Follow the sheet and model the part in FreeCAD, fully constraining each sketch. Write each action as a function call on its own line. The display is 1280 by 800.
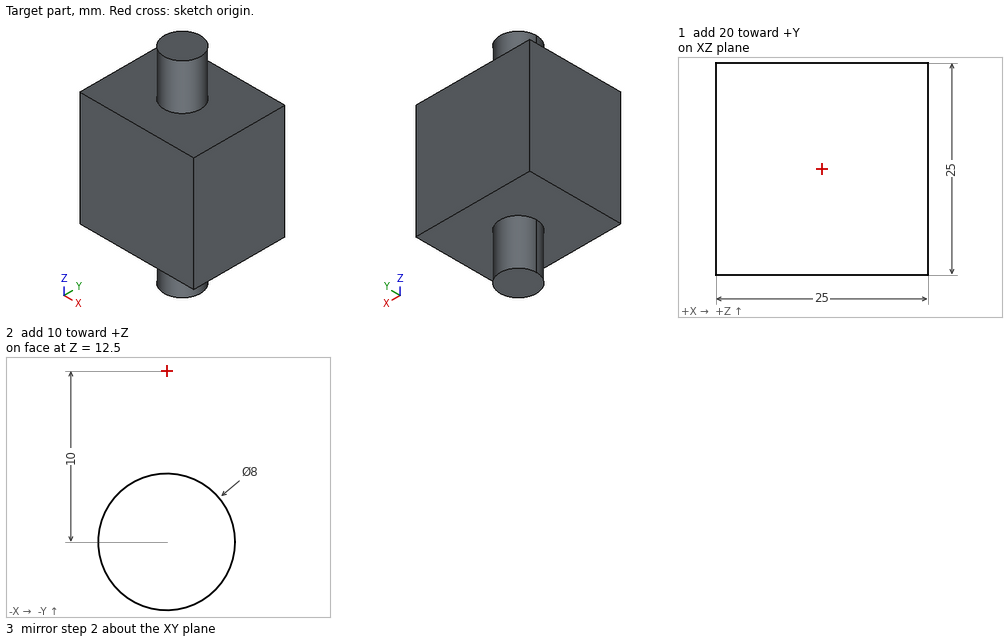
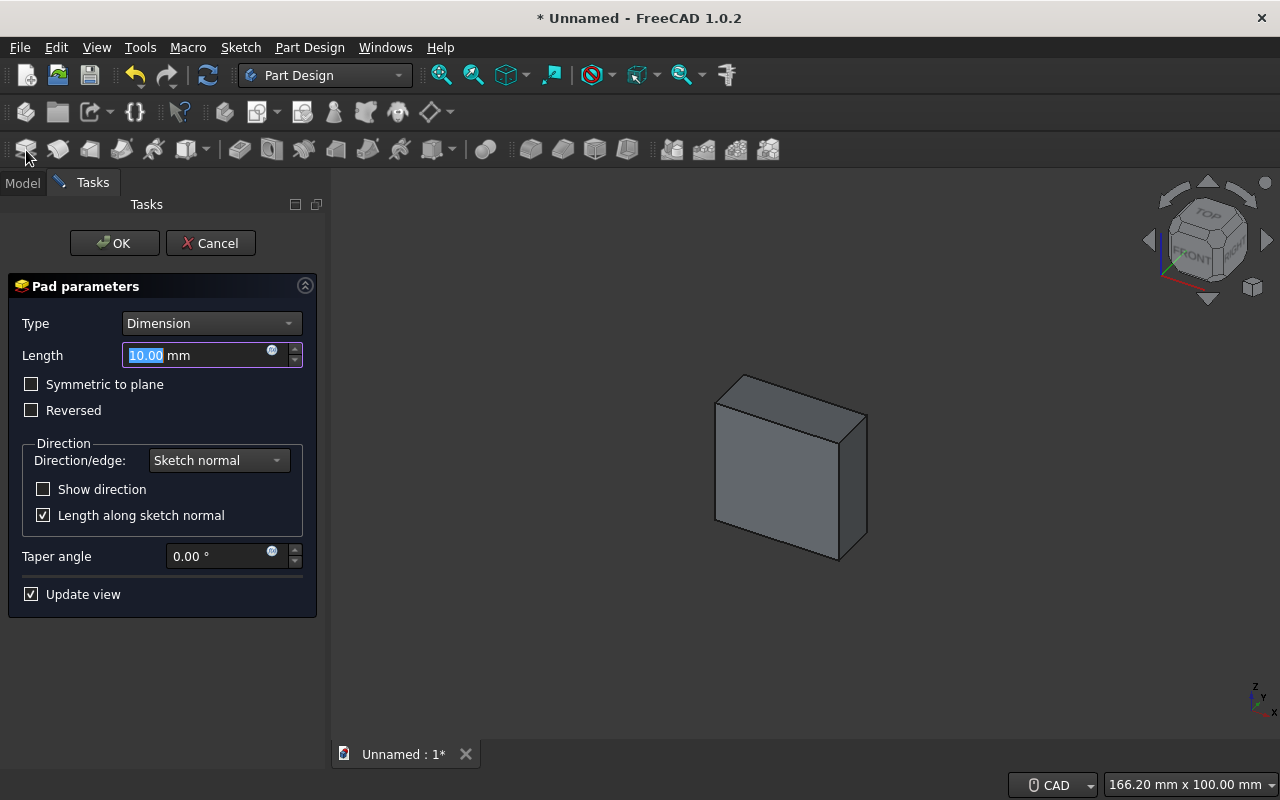
text(20)
key(Tab)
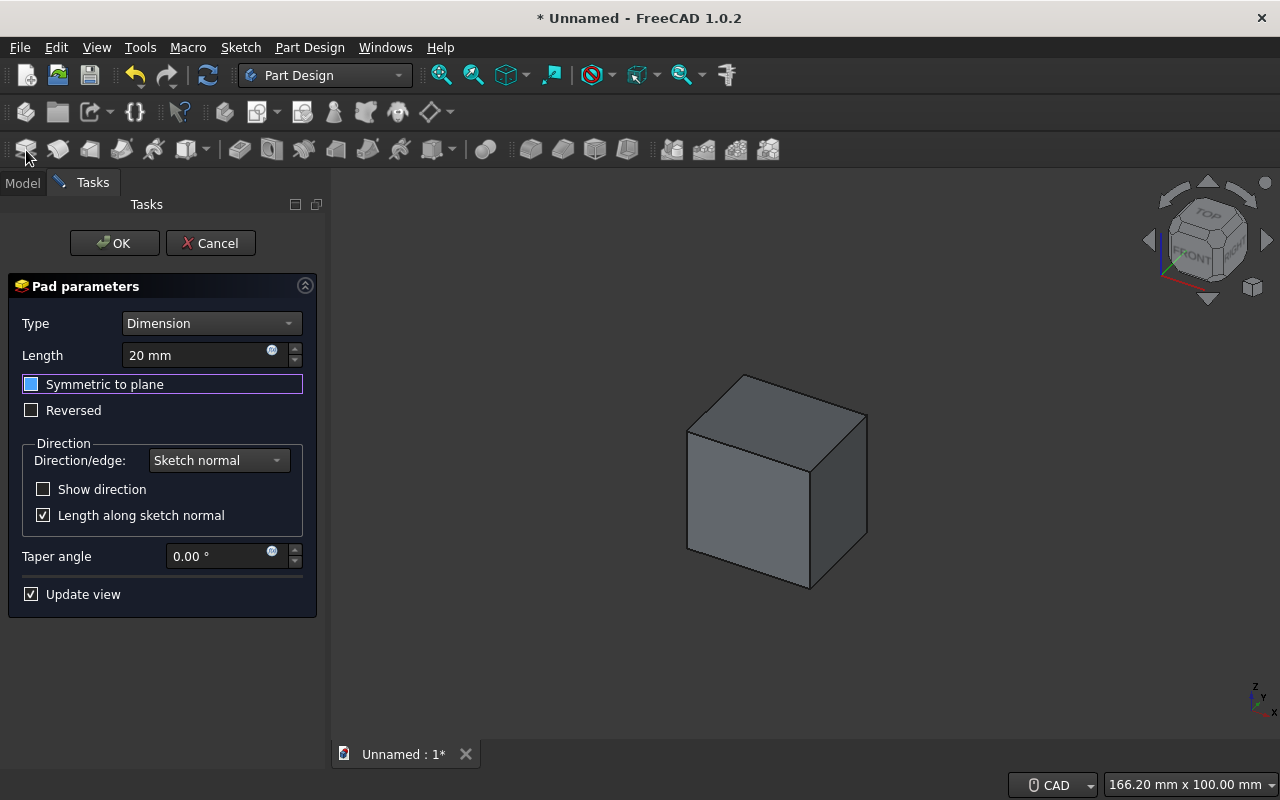
click(30, 410)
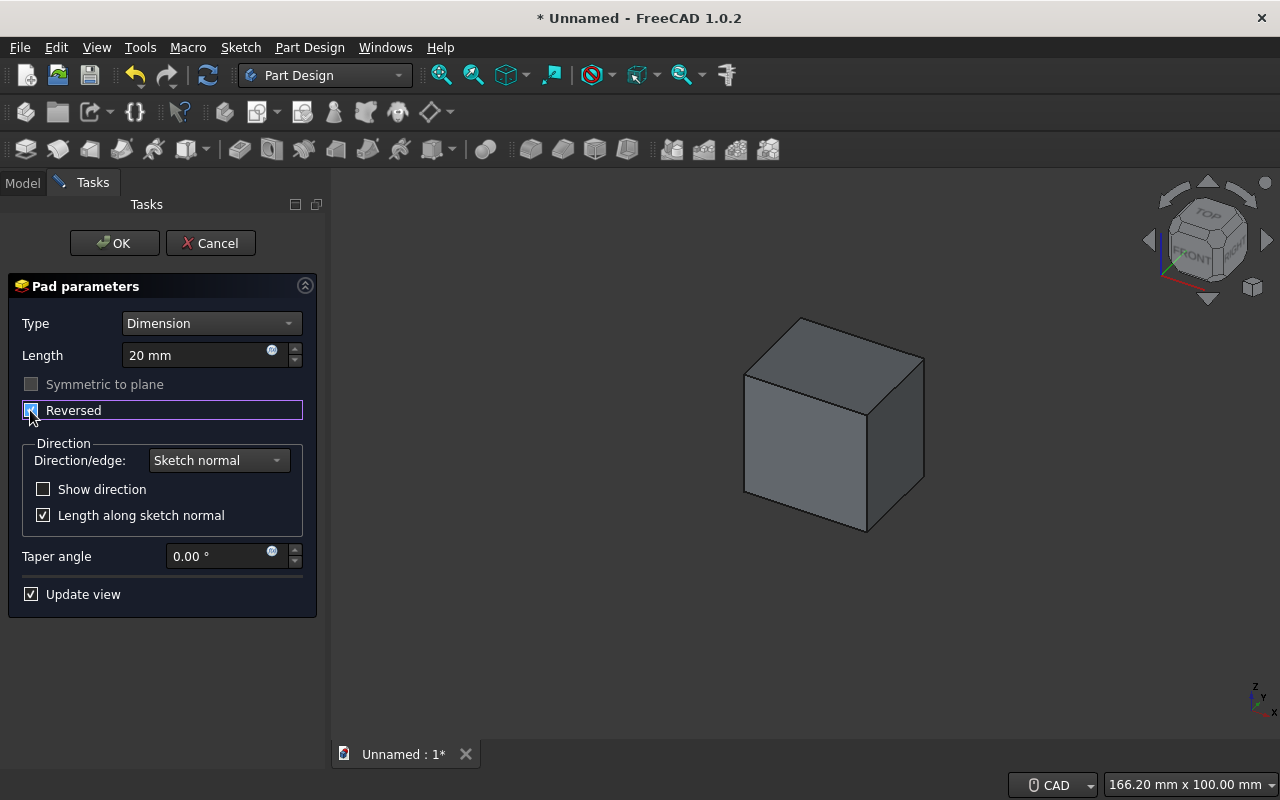
click(115, 243)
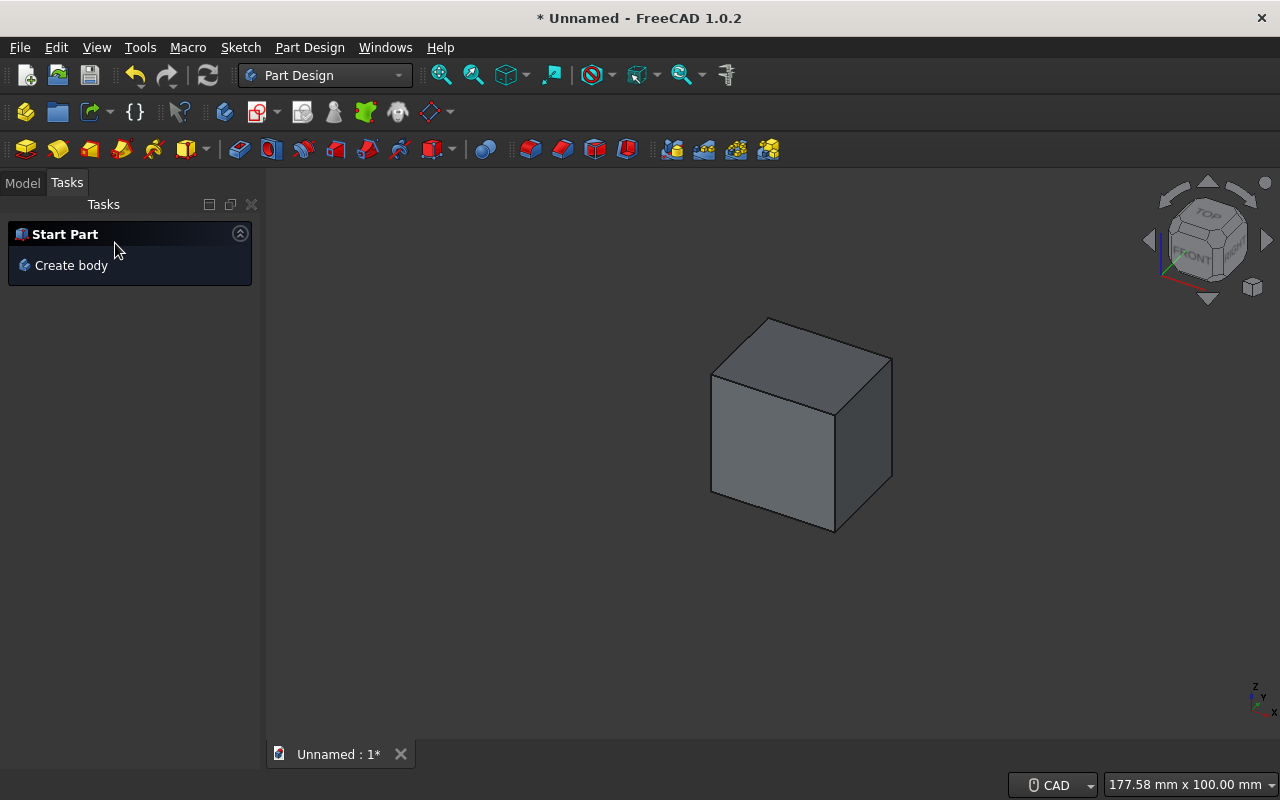
key(v)
key(f)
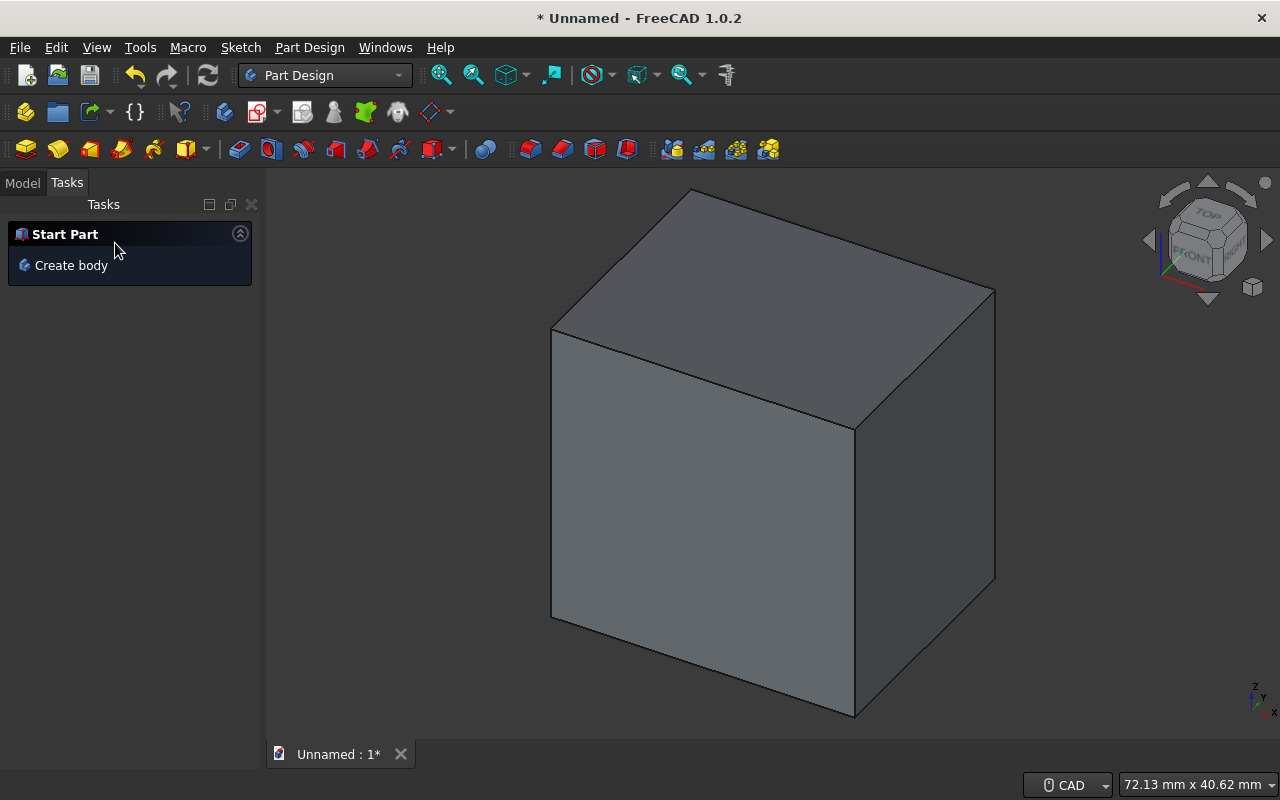
click(773, 309)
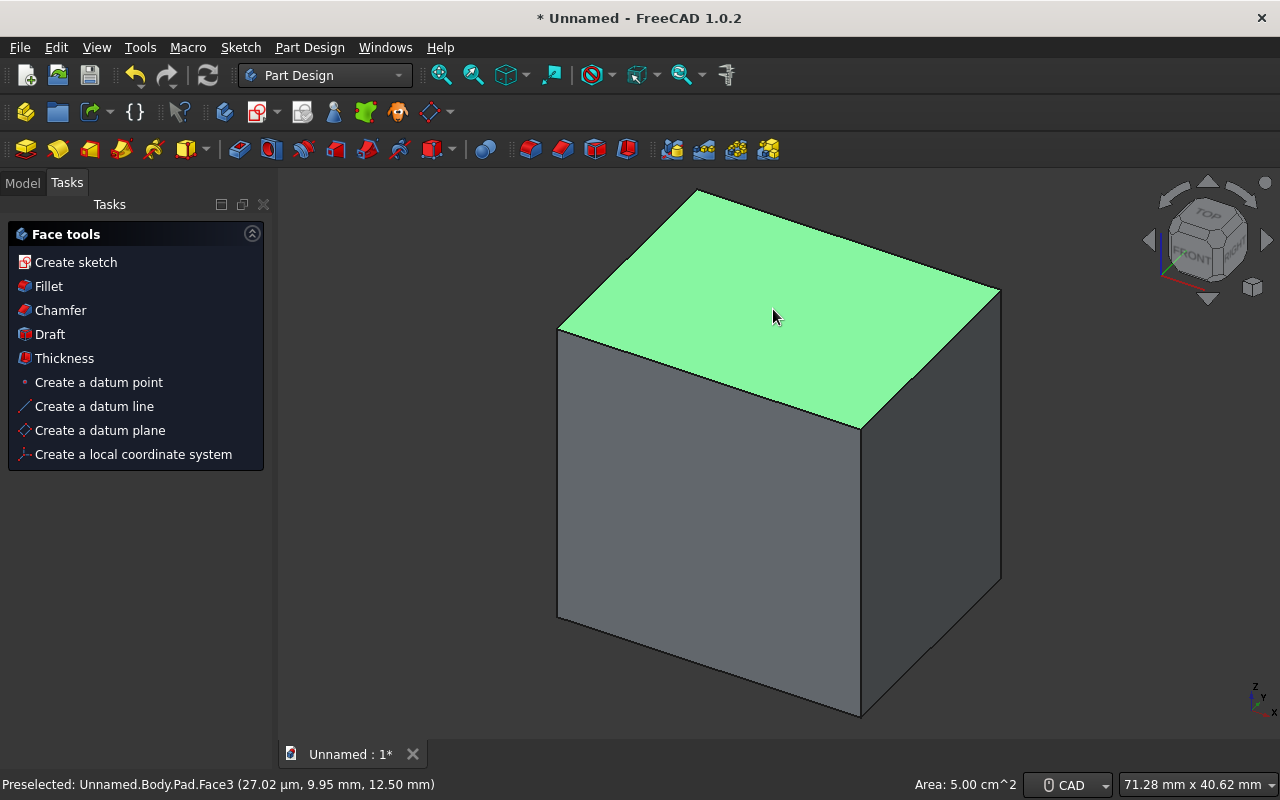
click(258, 112)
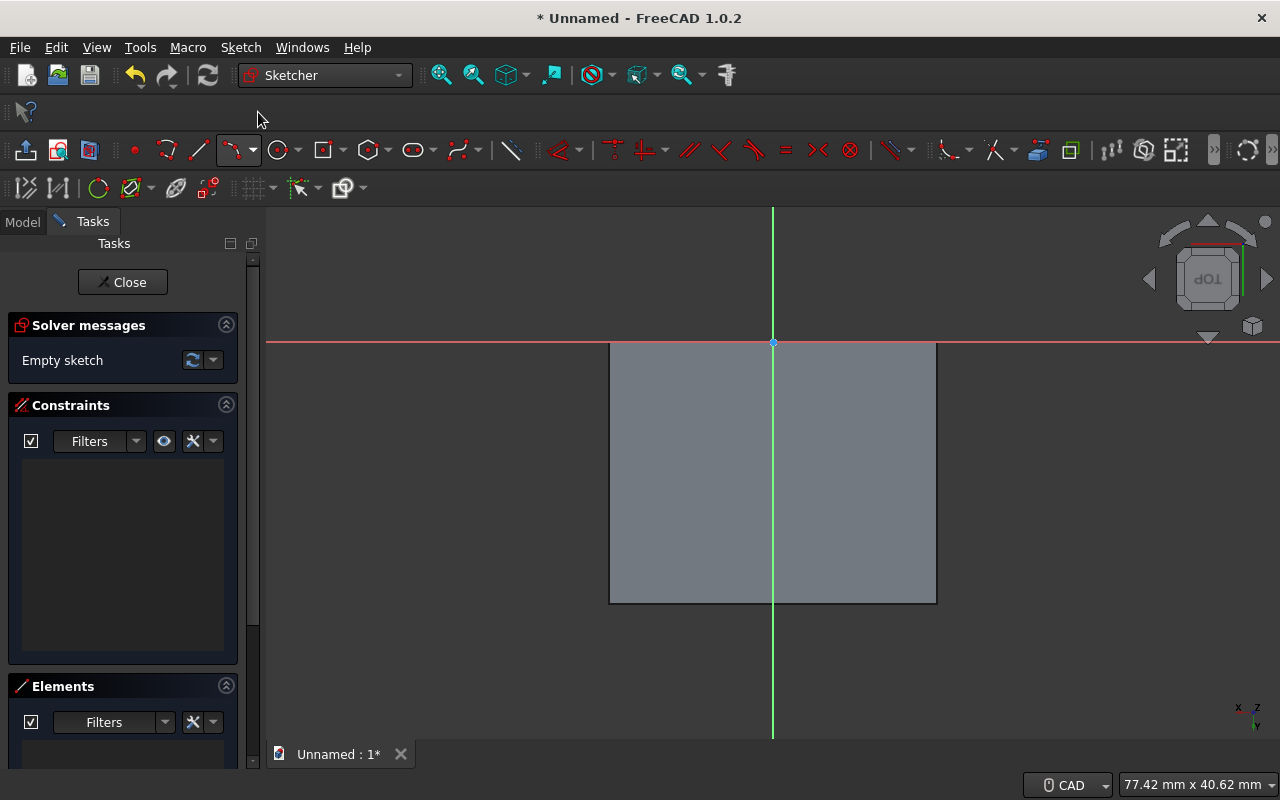
scroll(856, 386, up, 3)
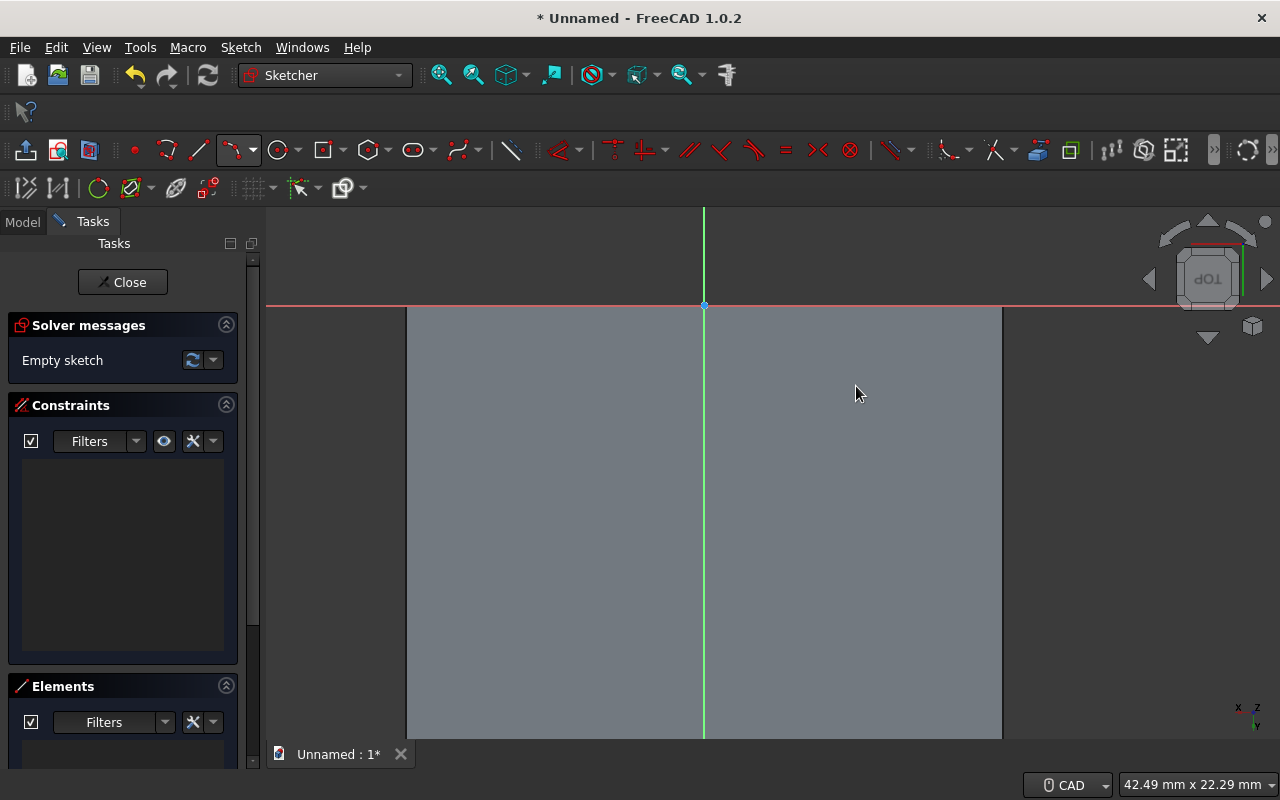
click(278, 150)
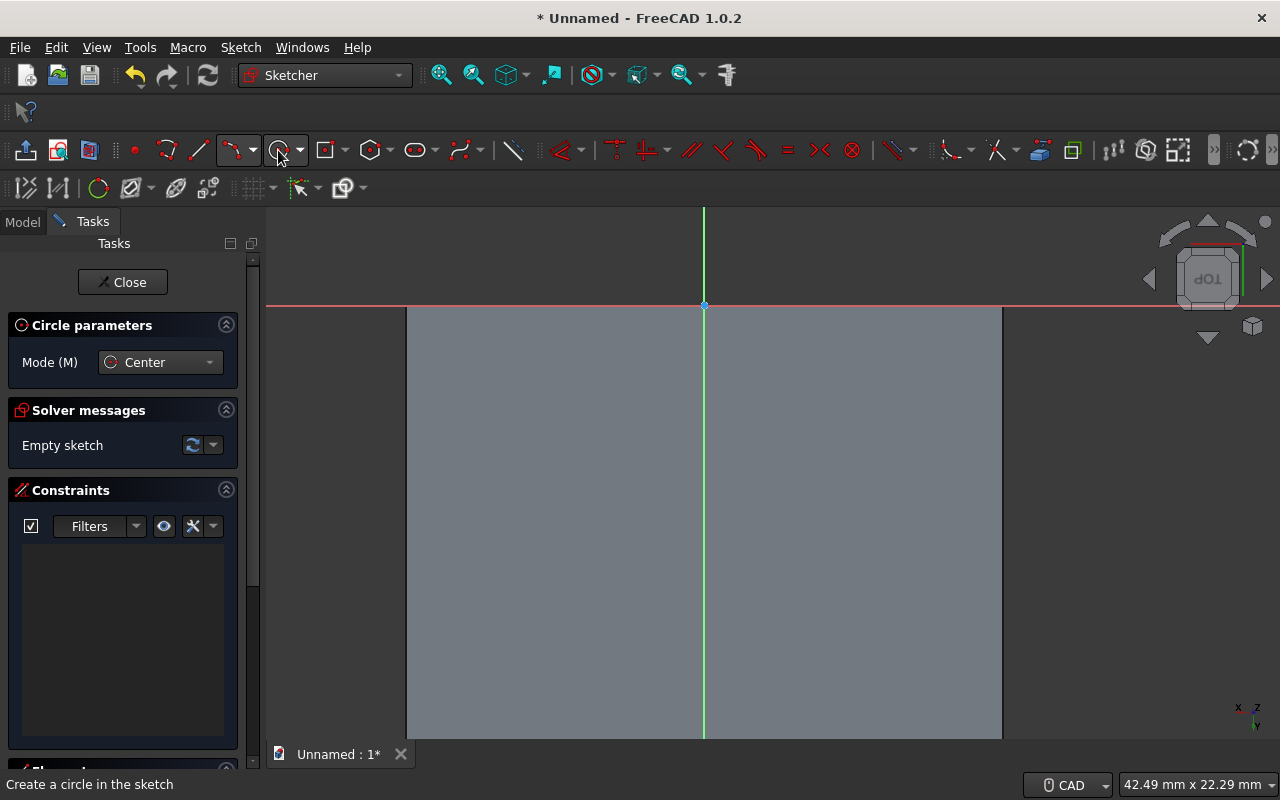
click(704, 544)
move(772, 477)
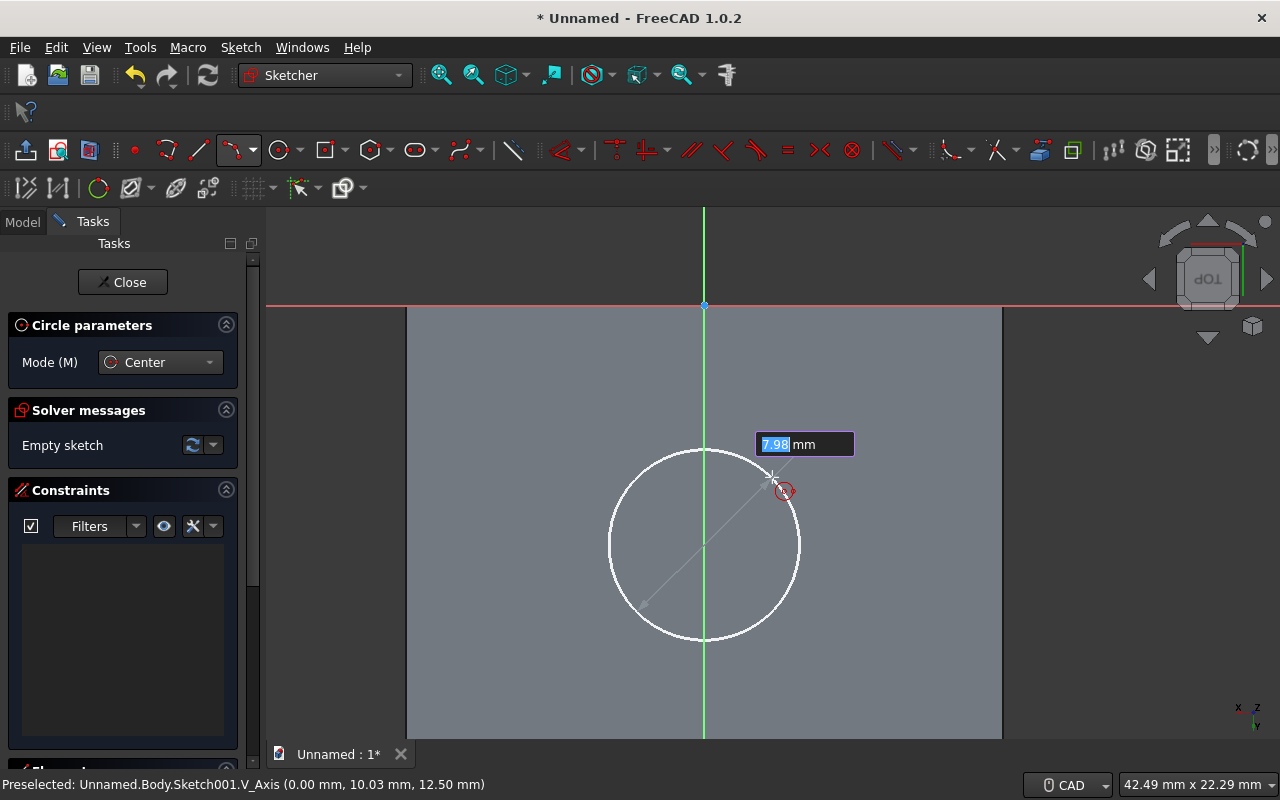
text(8)
key(Return)
key(Escape)